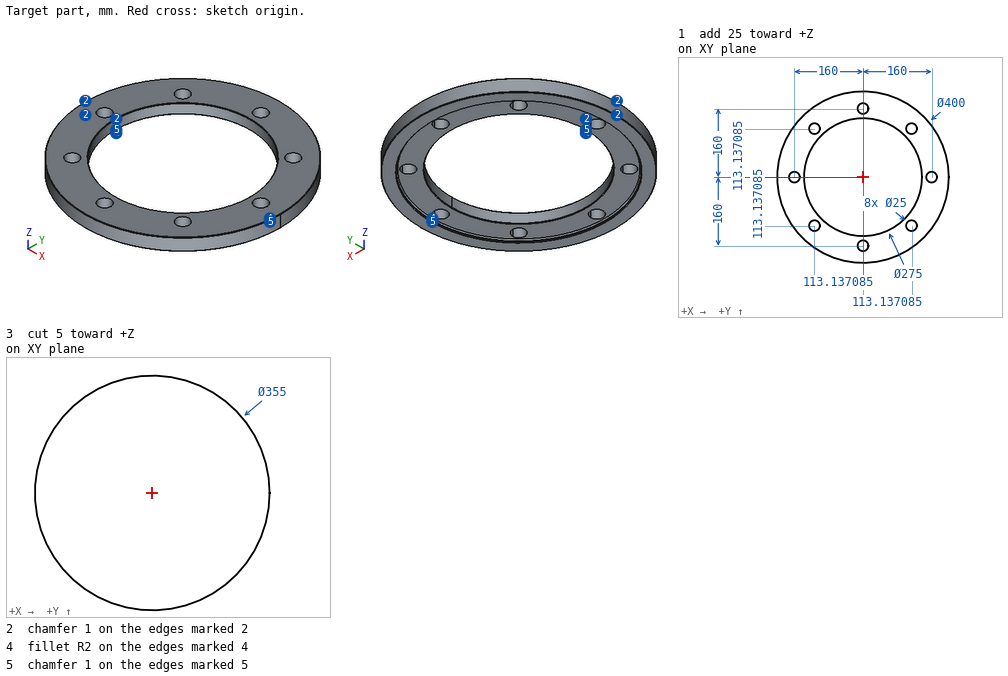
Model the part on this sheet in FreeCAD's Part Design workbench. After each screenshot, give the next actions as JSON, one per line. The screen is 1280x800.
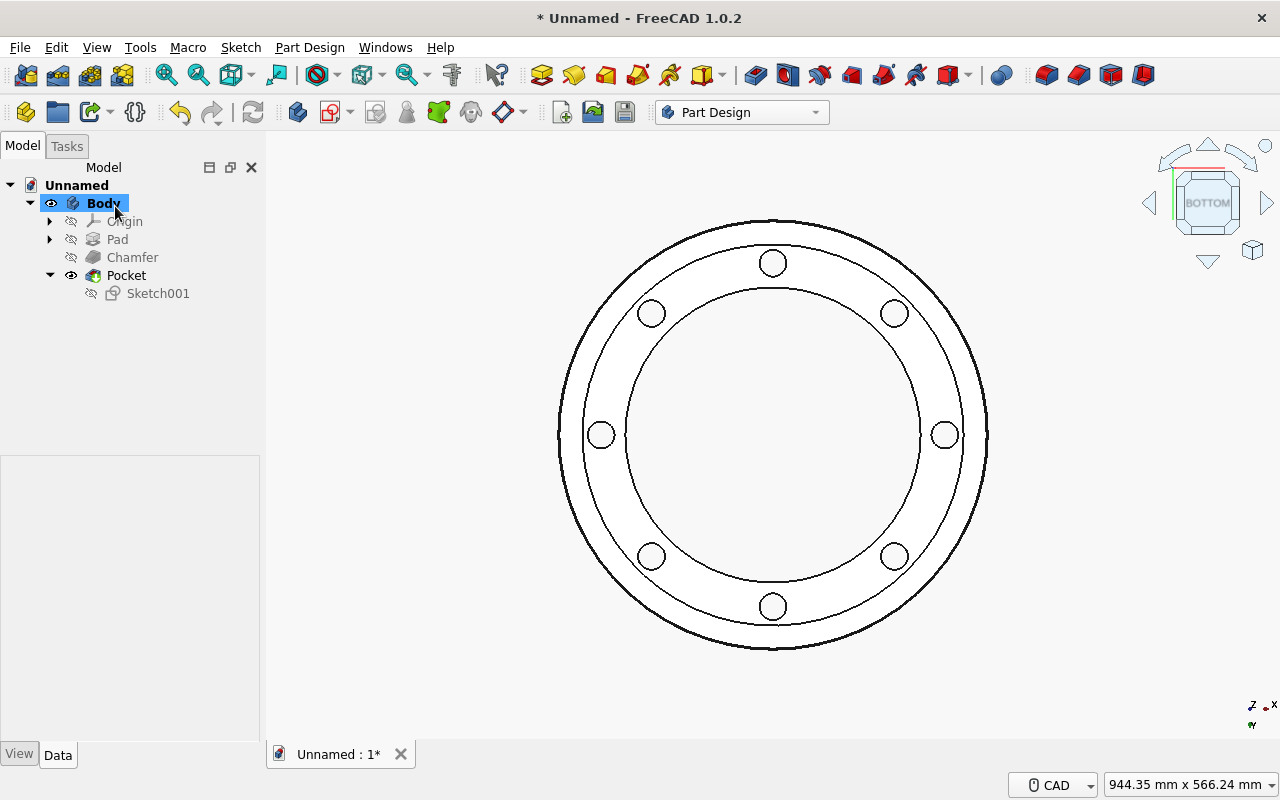
{"action": "key", "text": "0"}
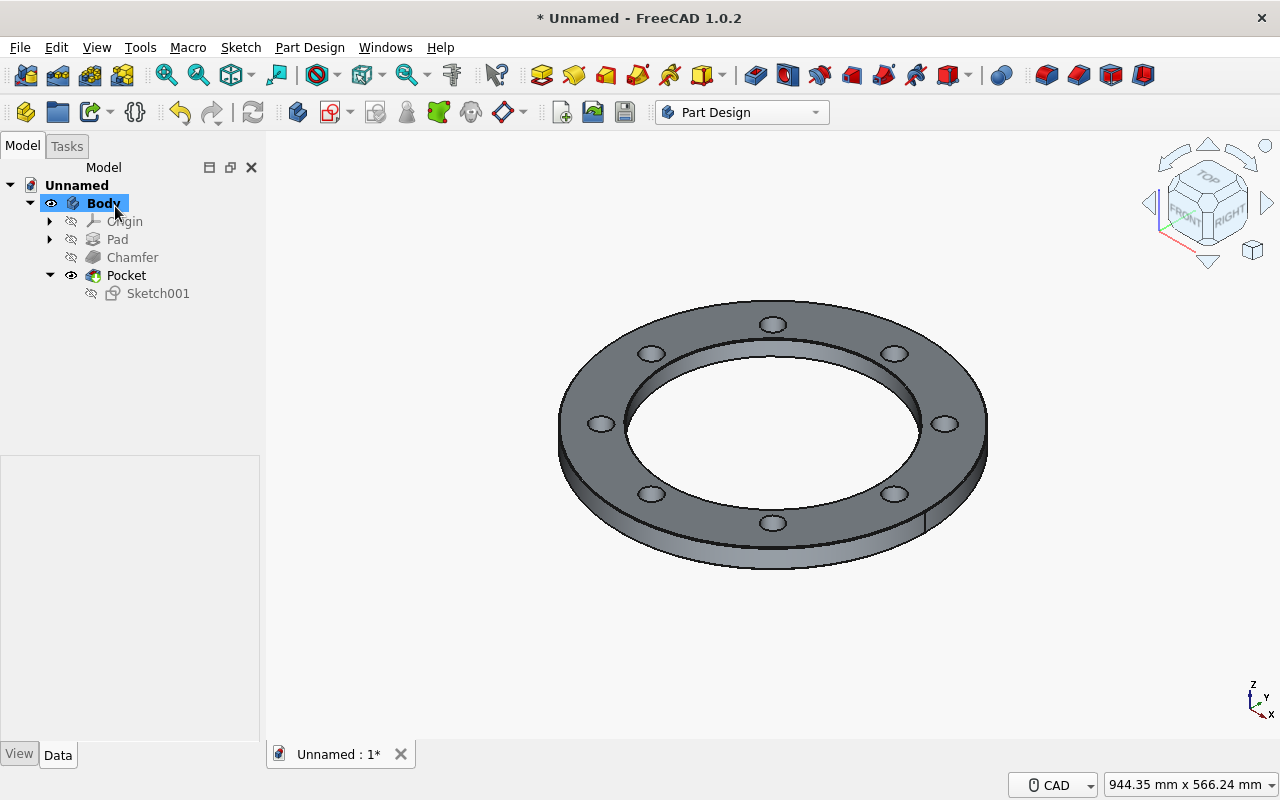
{"action": "key", "text": "2"}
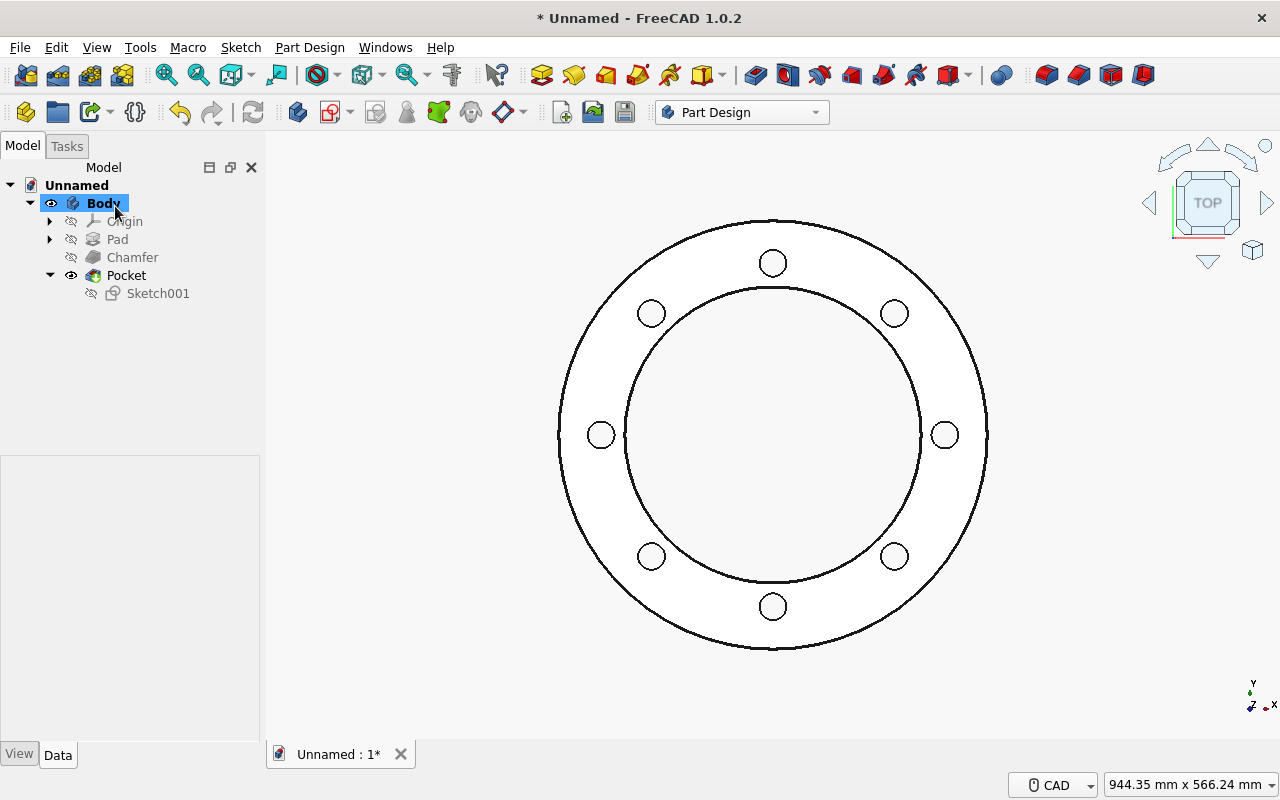
{"action": "key", "text": "1"}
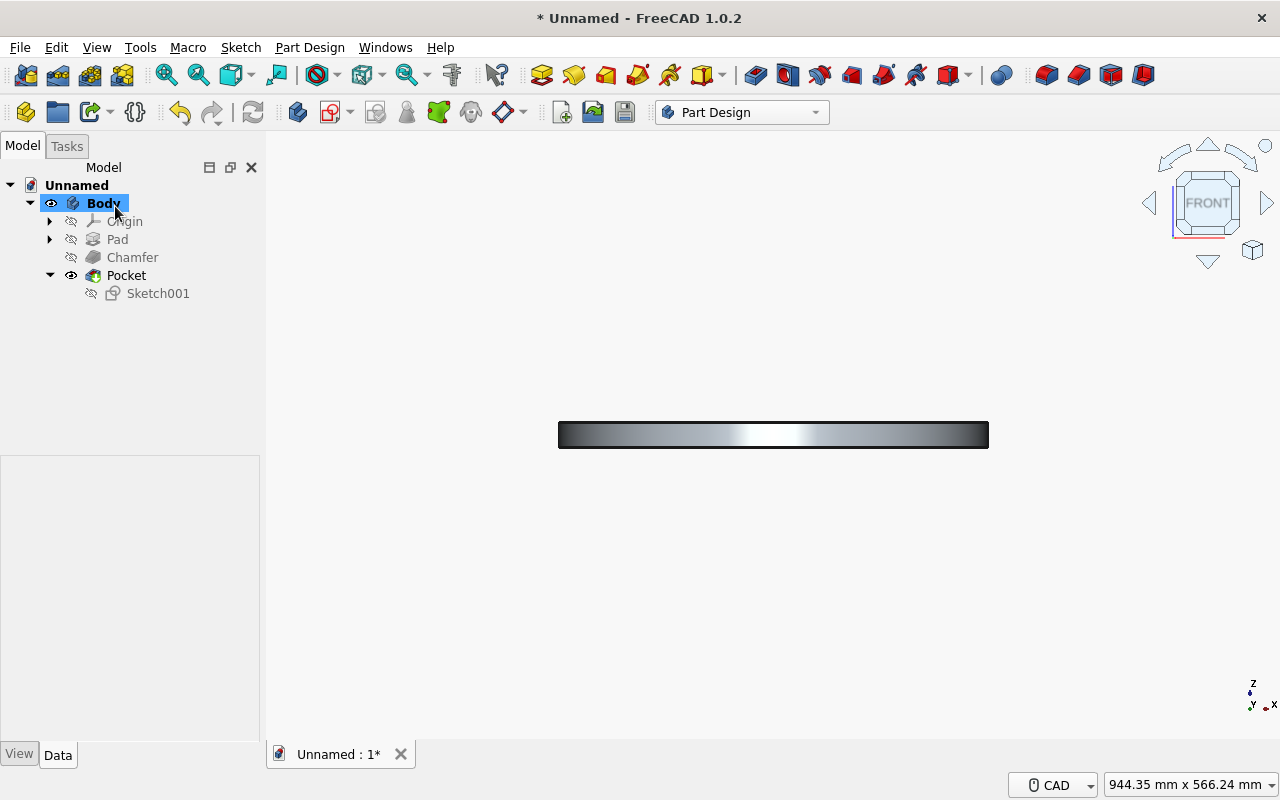
{"action": "left_click", "coordinate": [168, 76]}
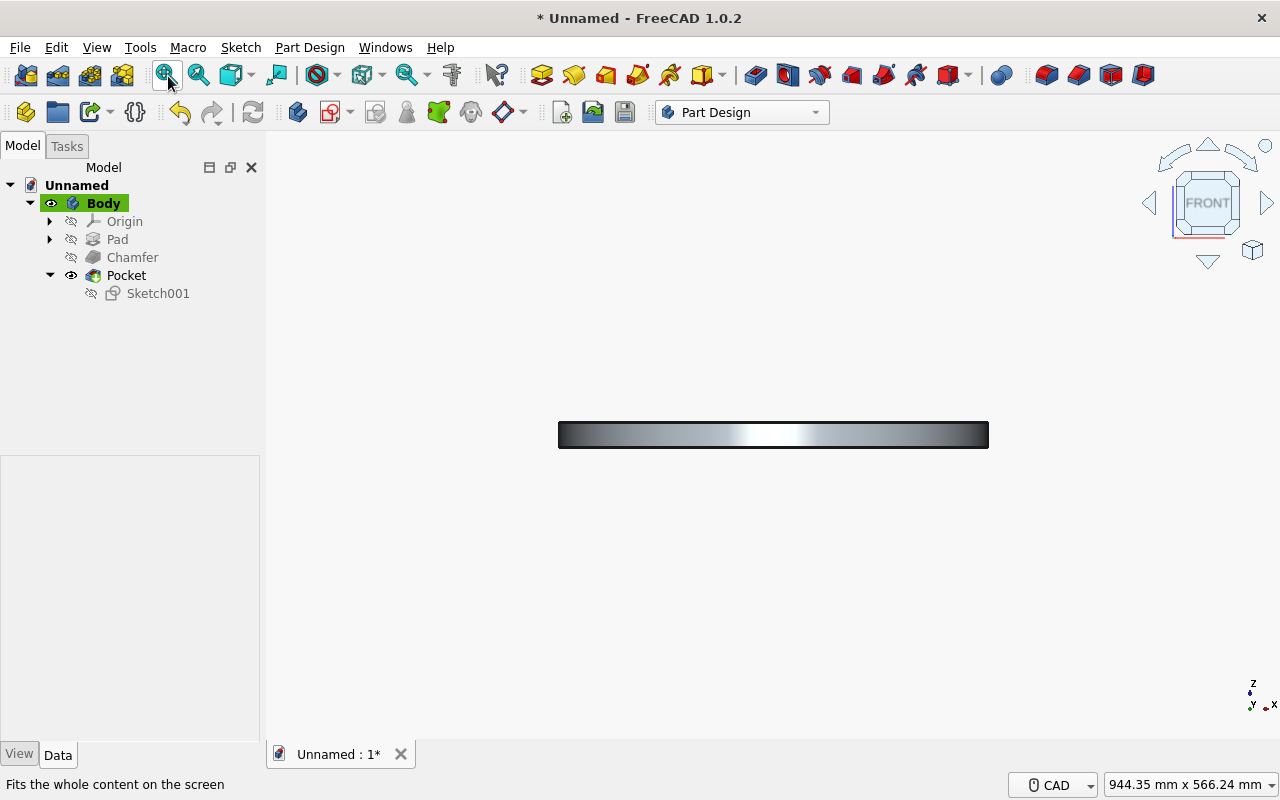
{"action": "key", "text": "3"}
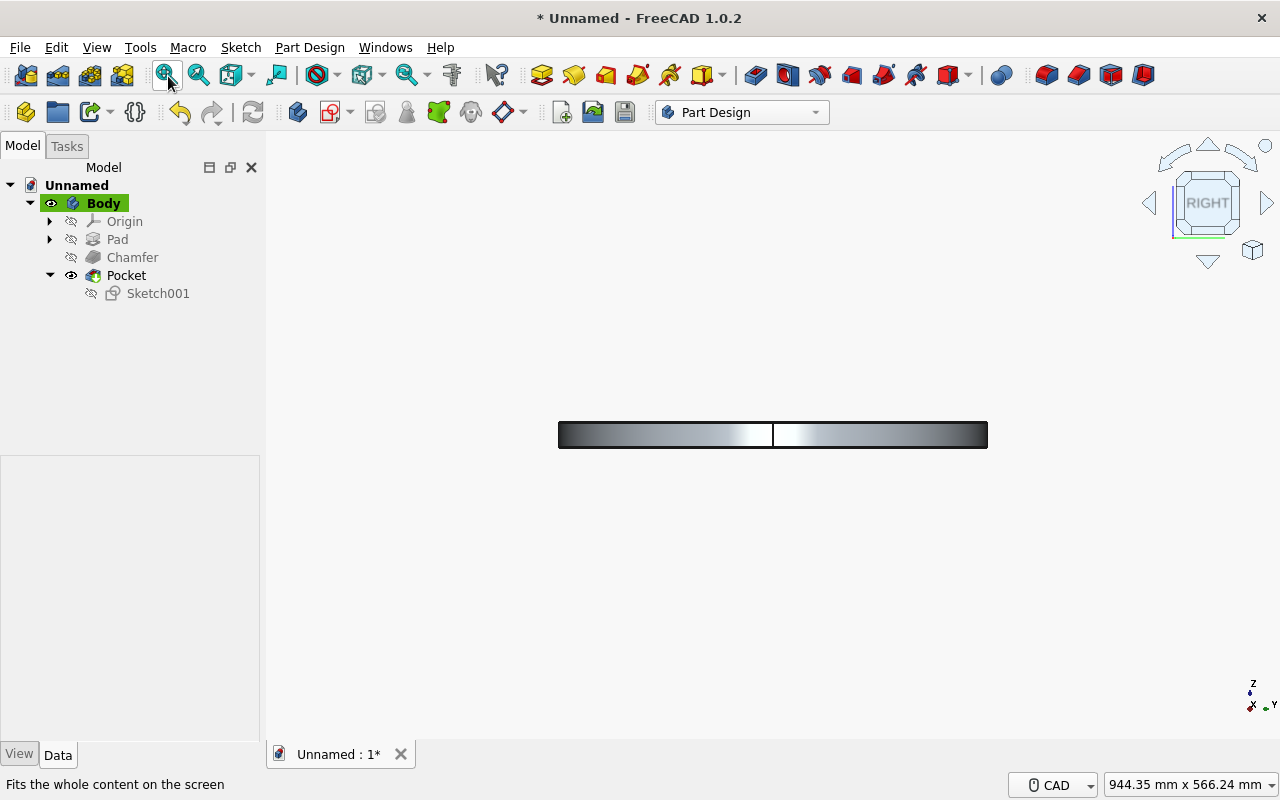
{"action": "left_click", "coordinate": [168, 76]}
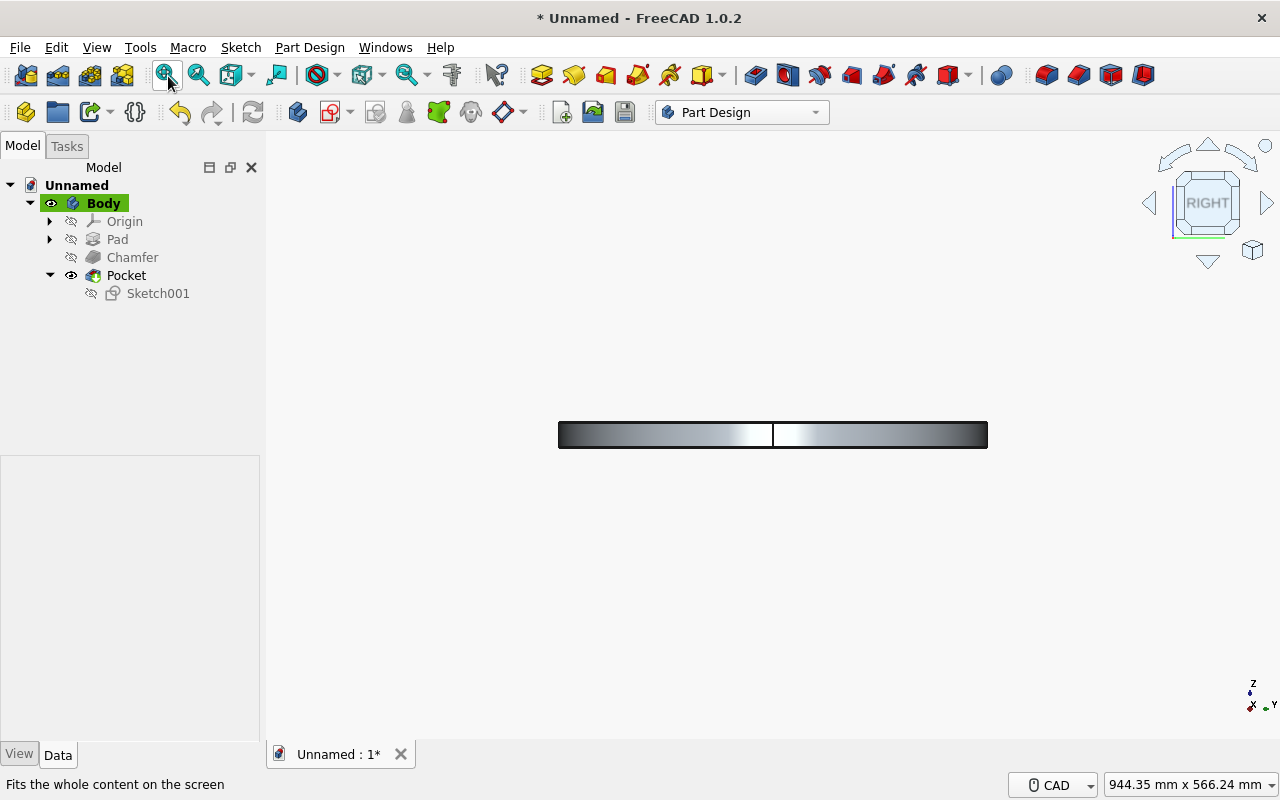
{"action": "key", "text": "5"}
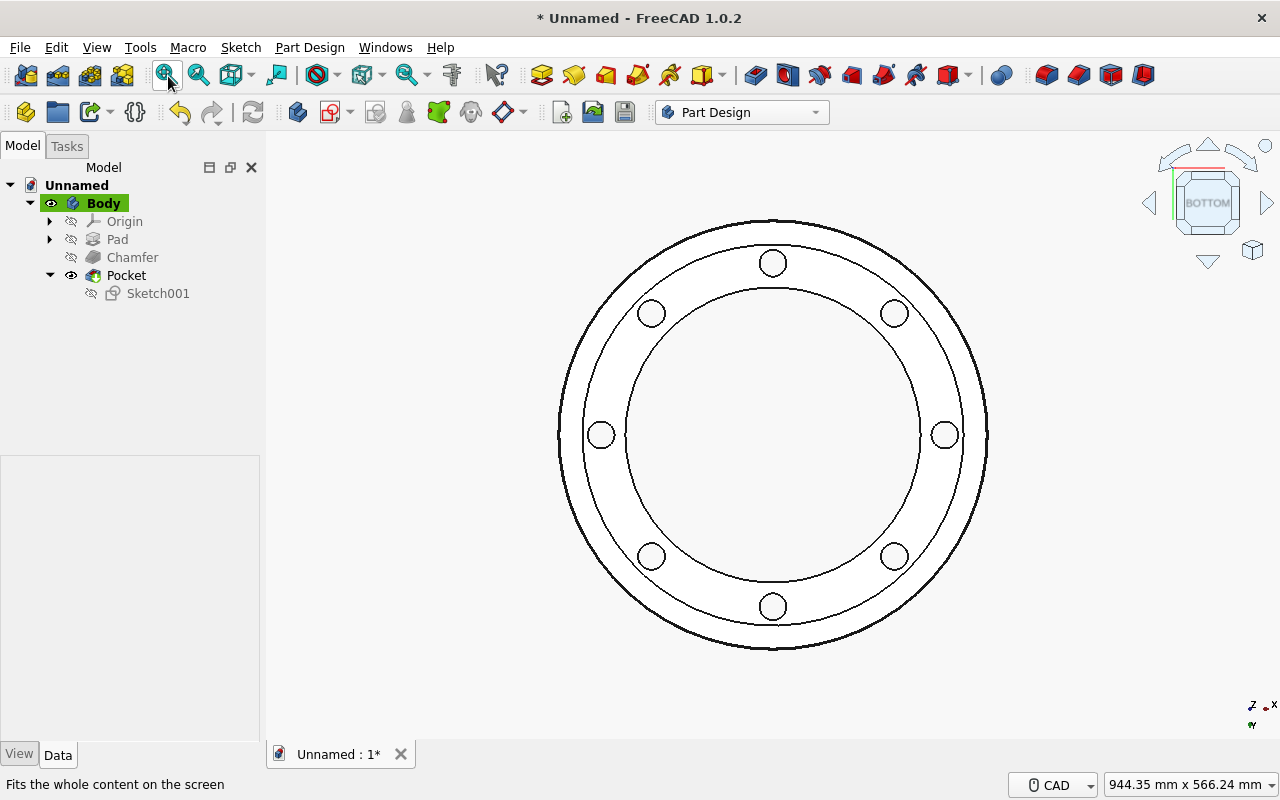
{"action": "key", "text": "4"}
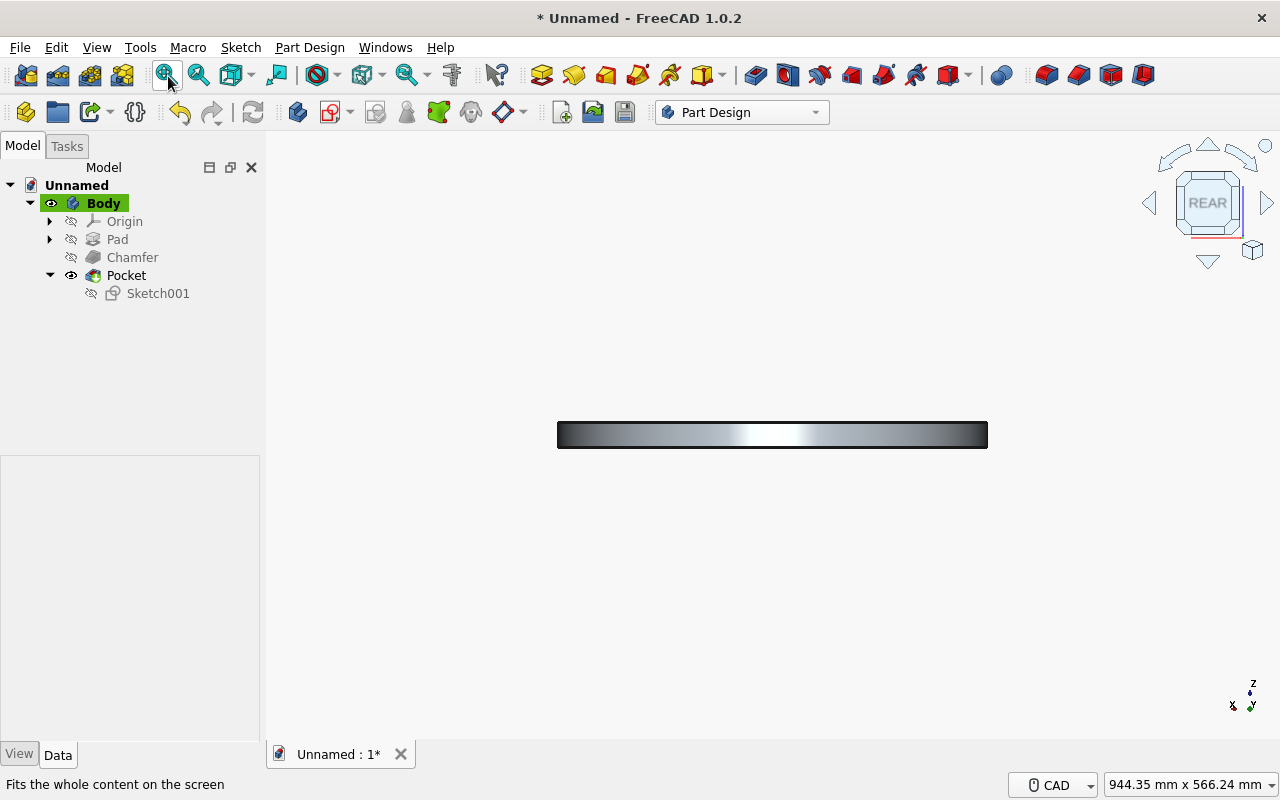
{"action": "left_click", "coordinate": [168, 76]}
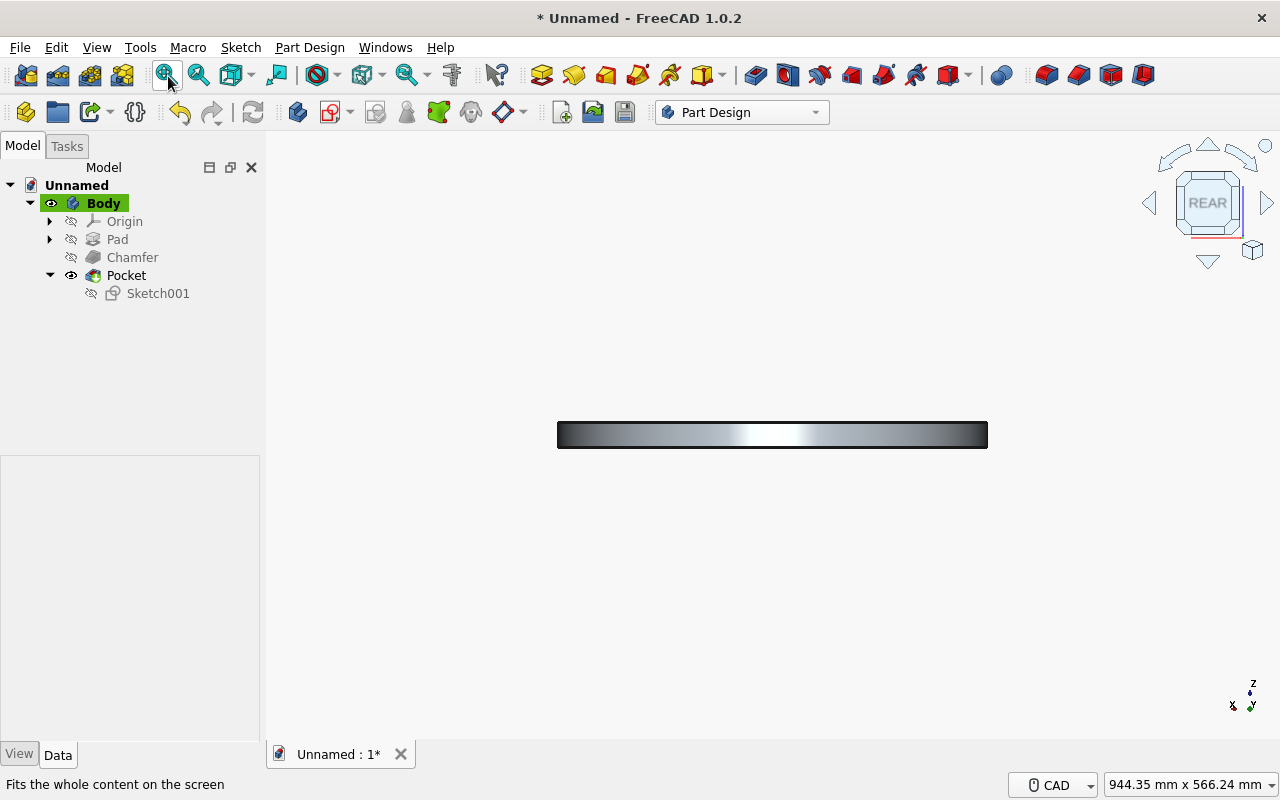
{"action": "key", "text": "6"}